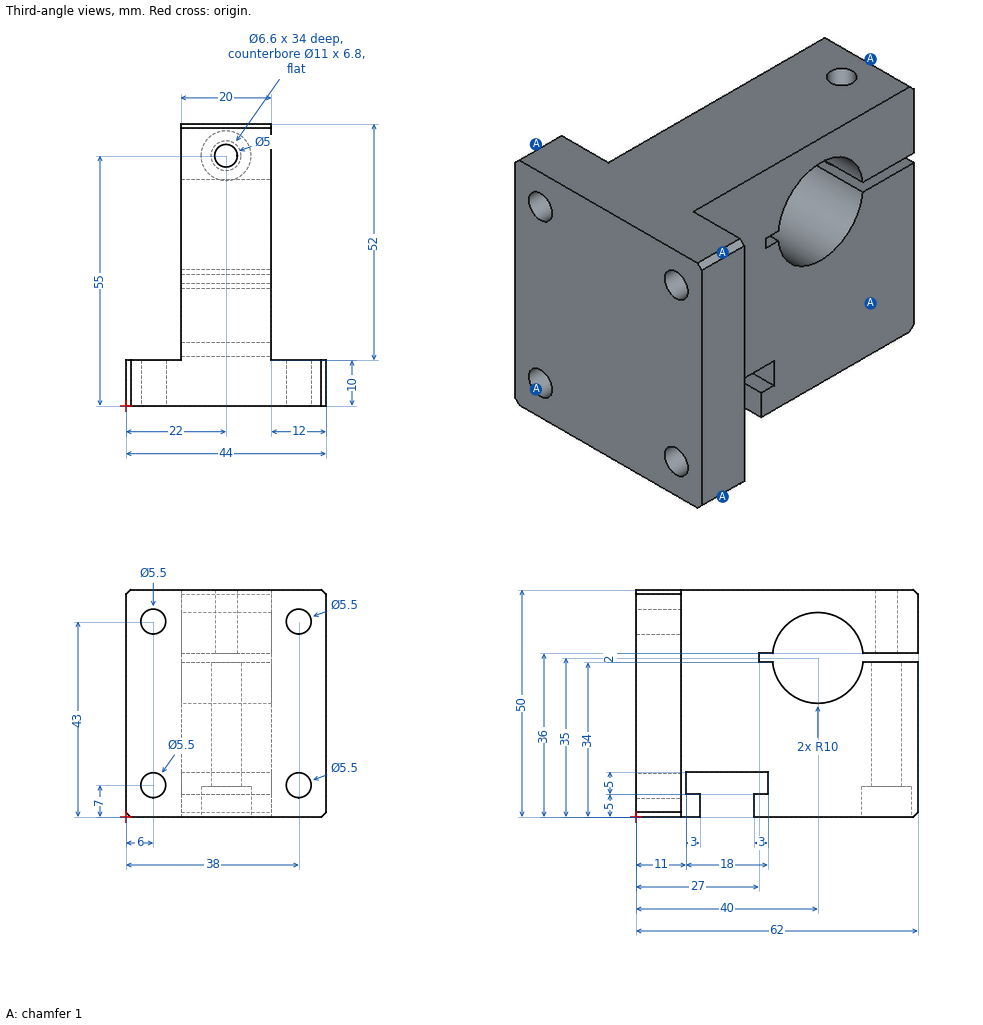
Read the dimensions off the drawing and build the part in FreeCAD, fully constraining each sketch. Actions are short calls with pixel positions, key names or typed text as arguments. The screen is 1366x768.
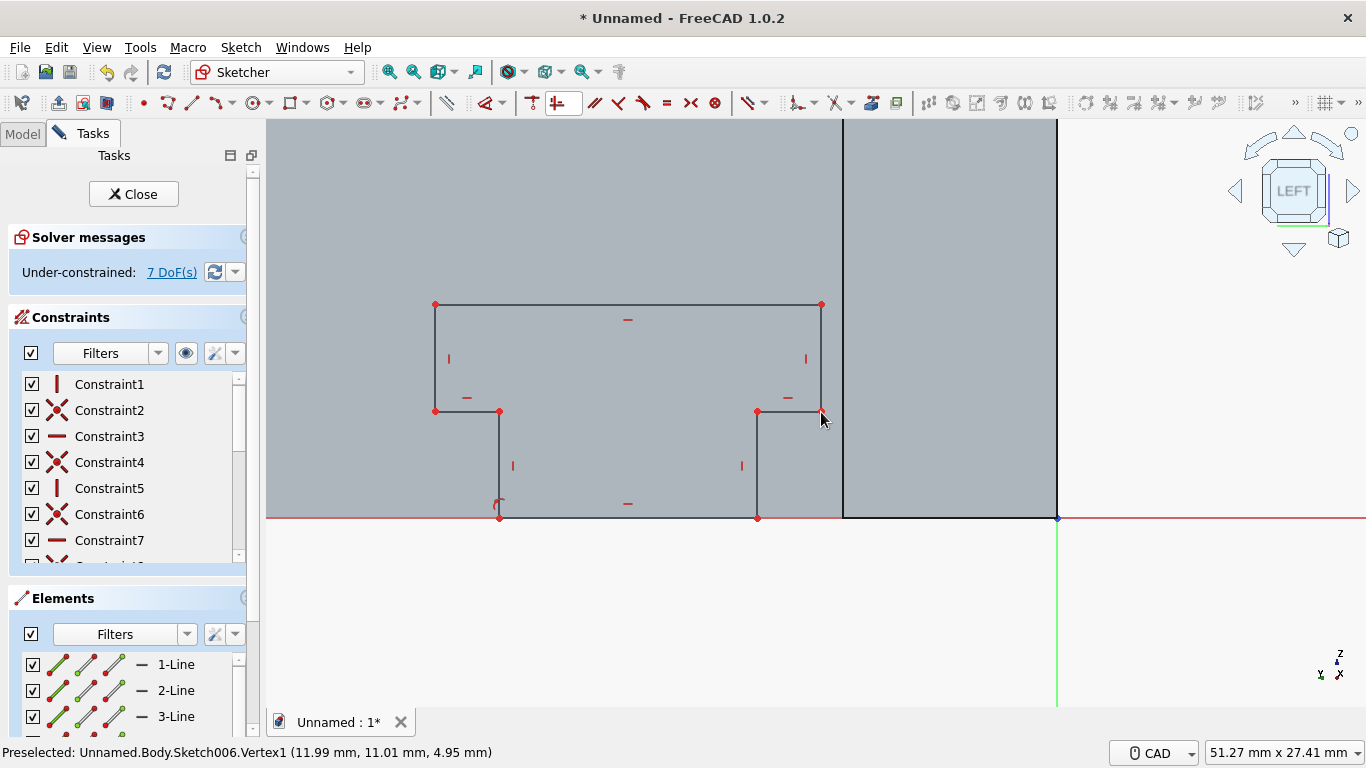
click(486, 104)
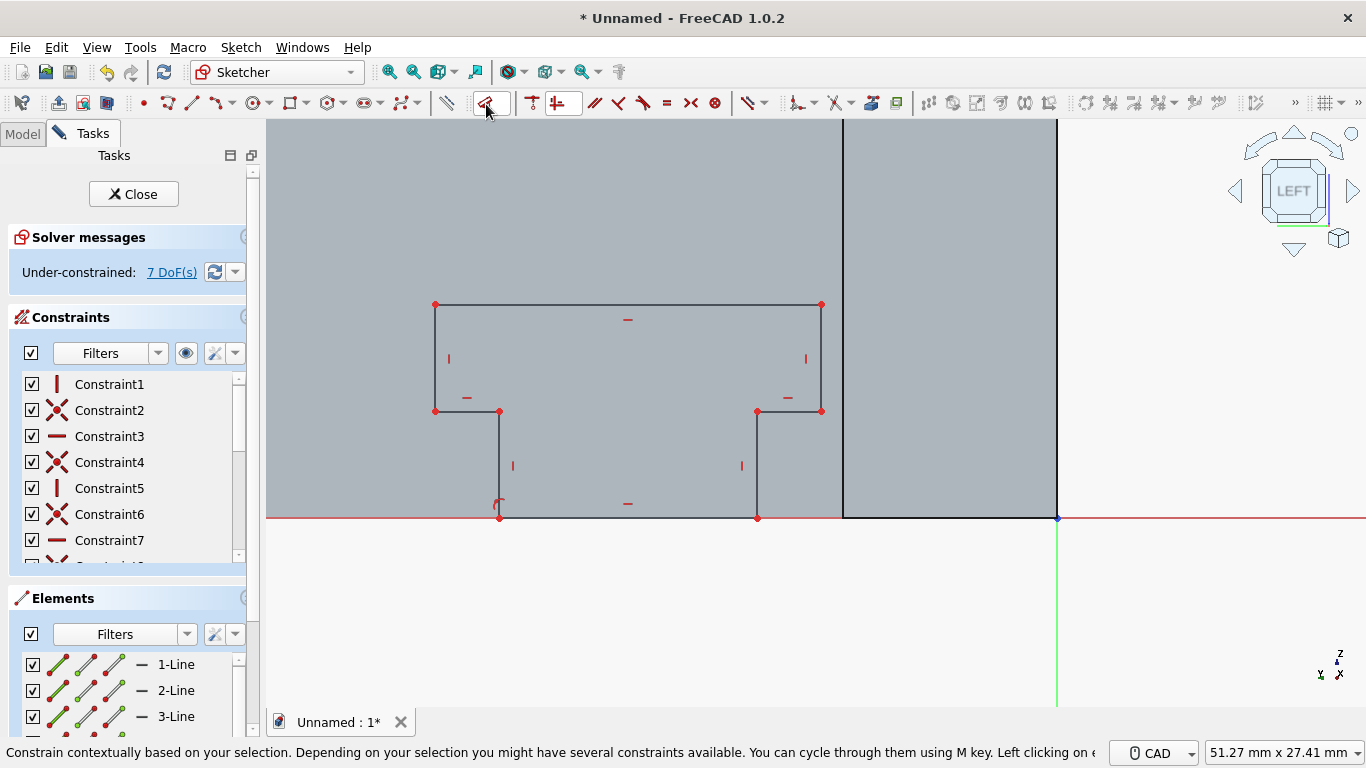
click(821, 380)
click(855, 358)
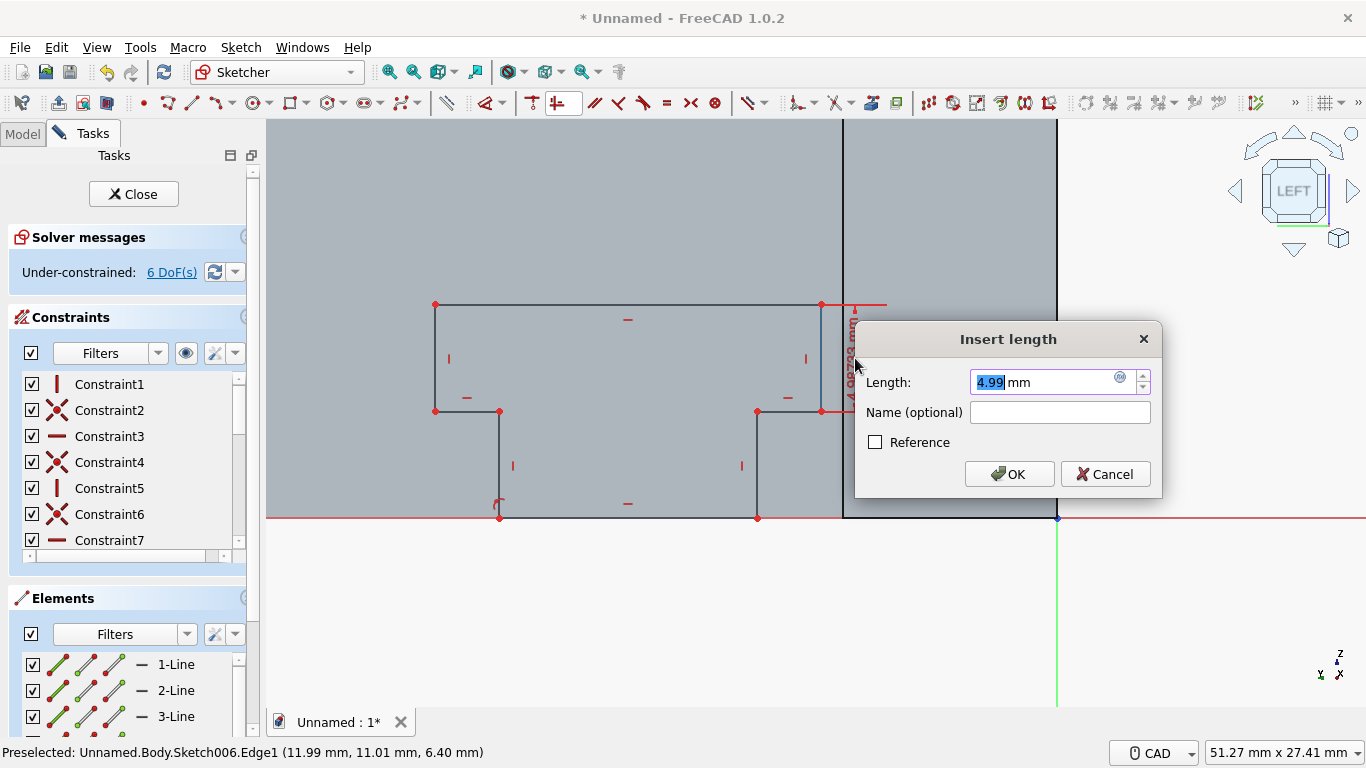
text(5)
key(Return)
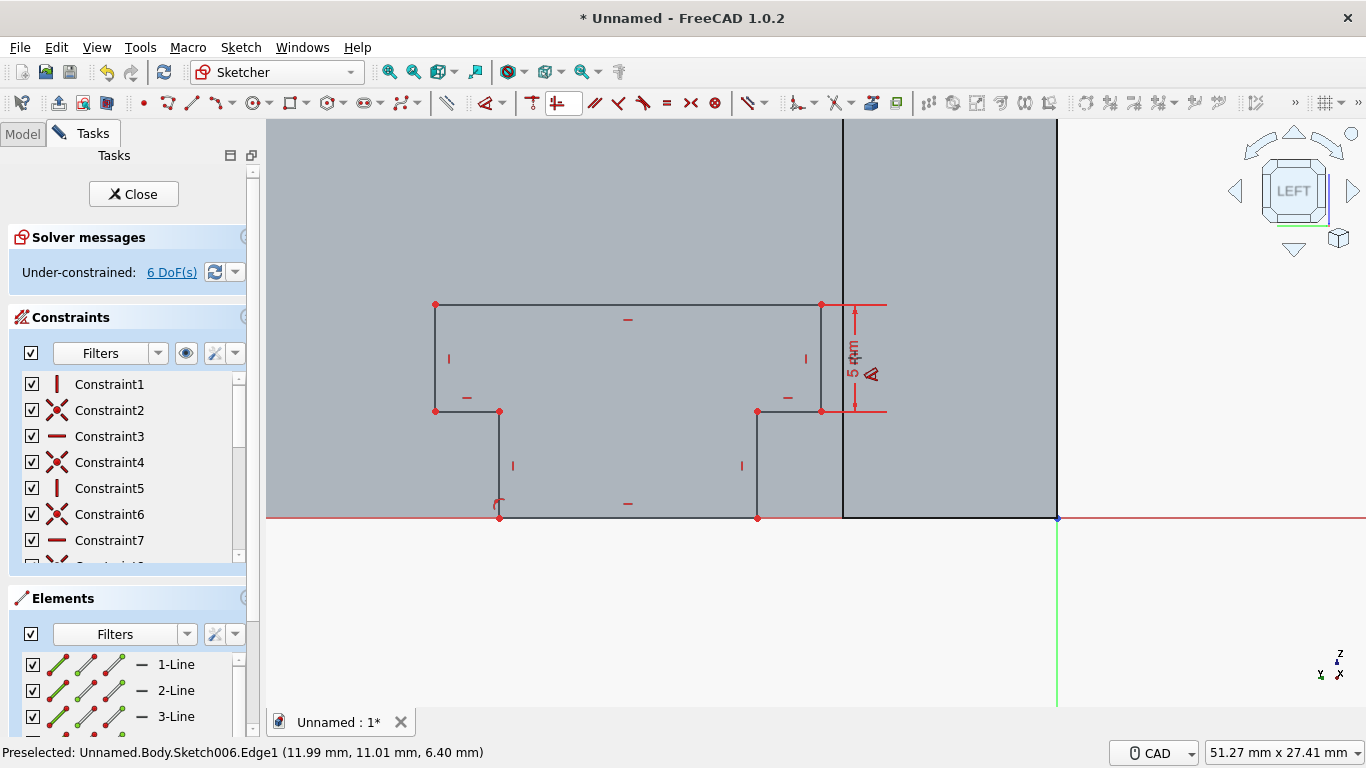
click(435, 337)
click(401, 358)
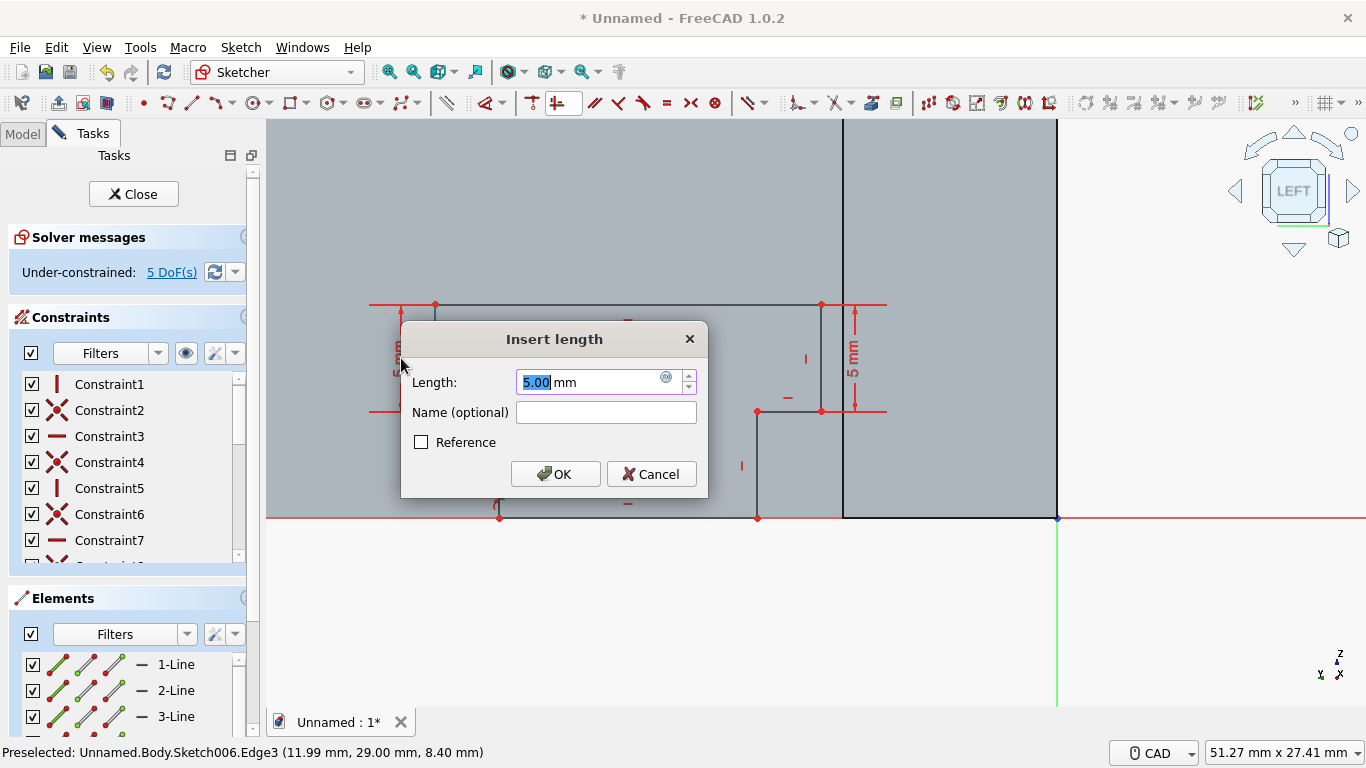
text(5)
key(Return)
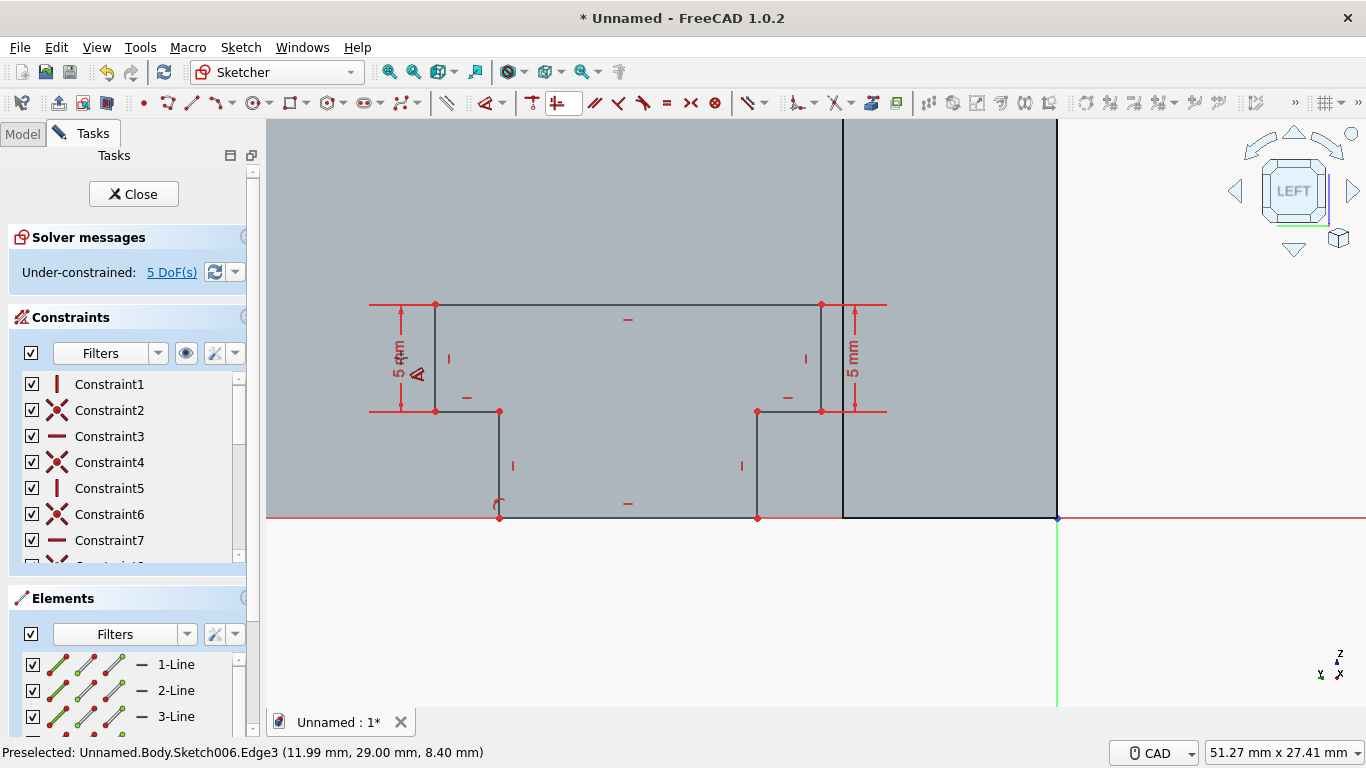
click(454, 412)
click(467, 446)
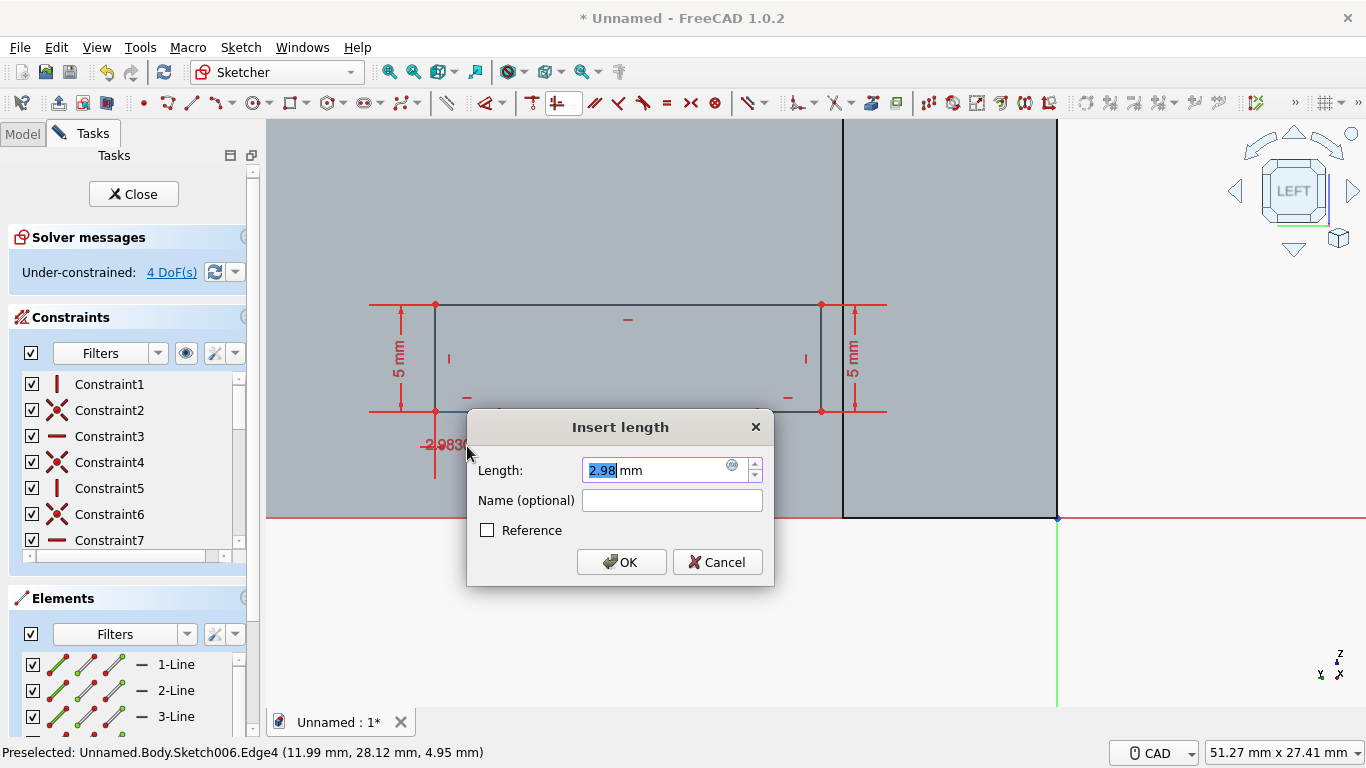
text(3)
key(Return)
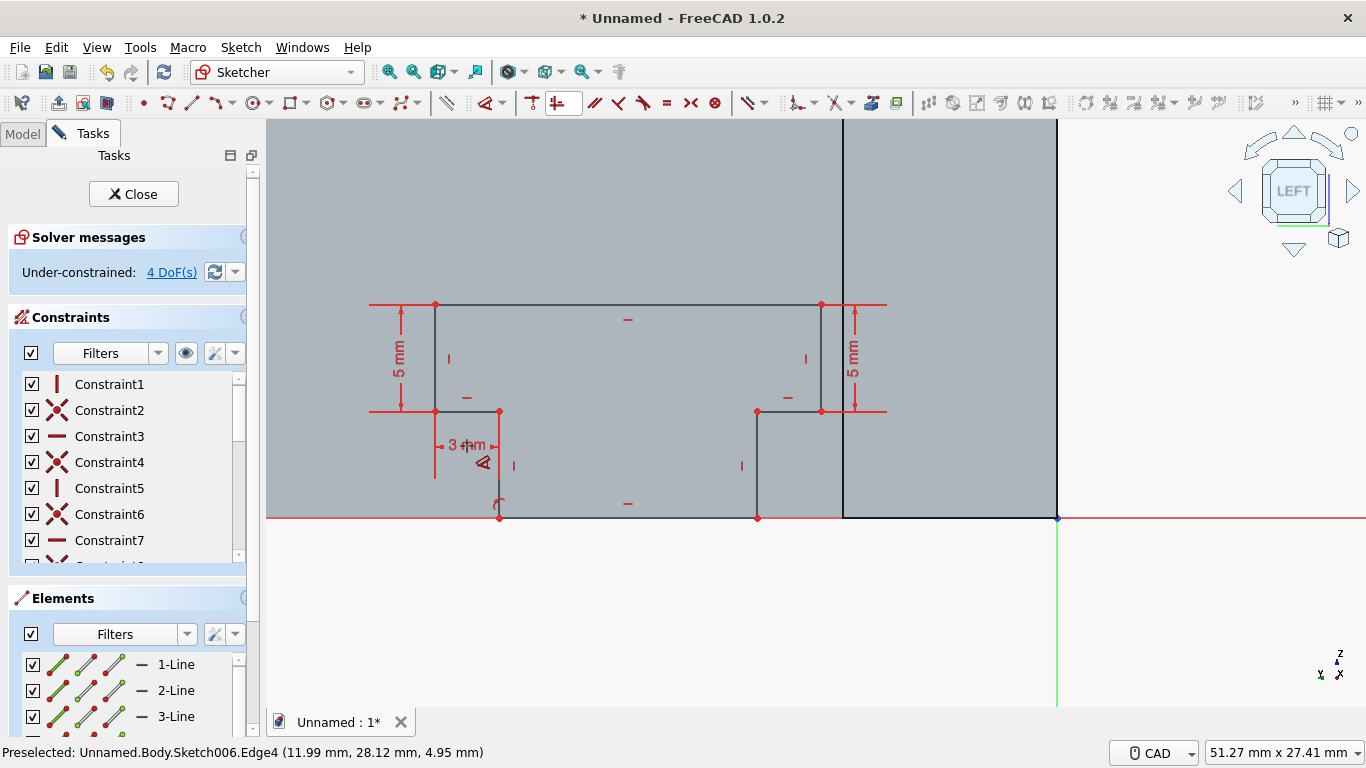
click(499, 444)
click(465, 490)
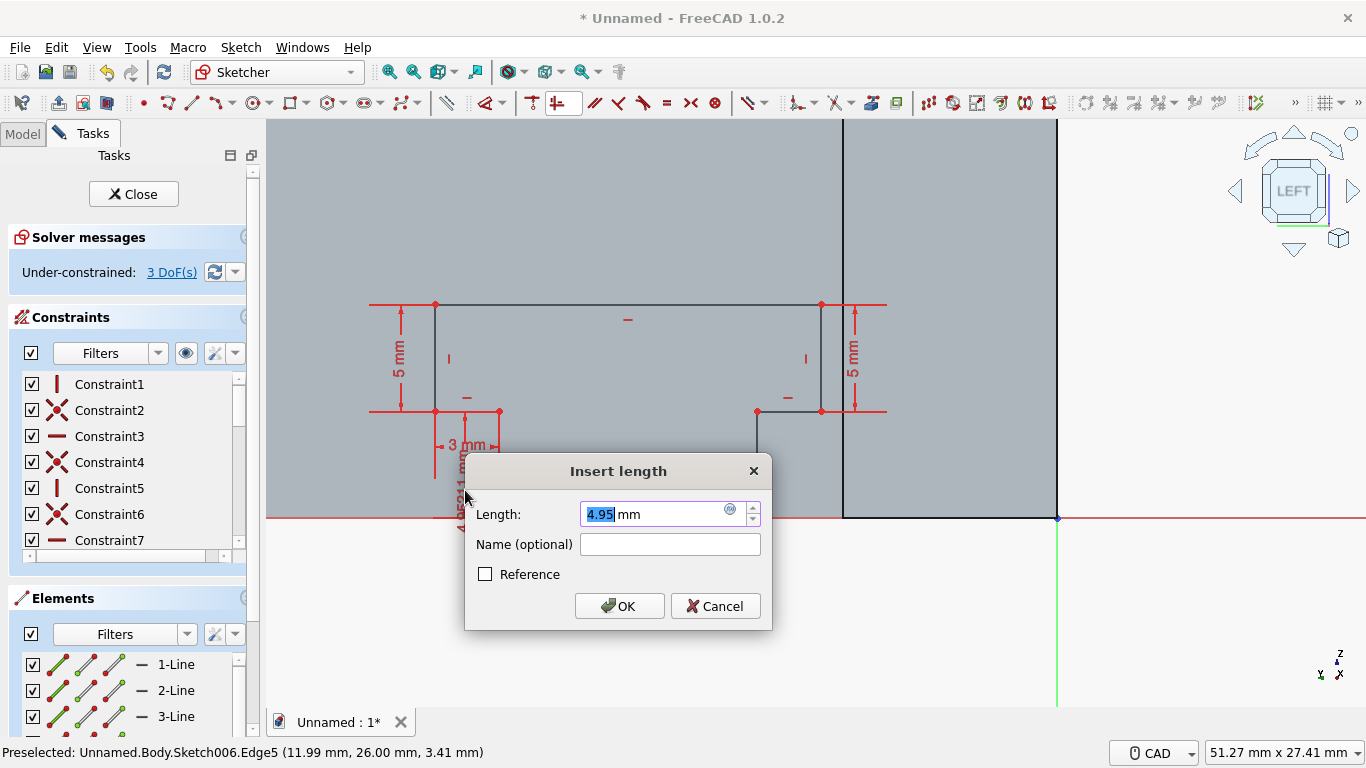
text(5)
key(Return)